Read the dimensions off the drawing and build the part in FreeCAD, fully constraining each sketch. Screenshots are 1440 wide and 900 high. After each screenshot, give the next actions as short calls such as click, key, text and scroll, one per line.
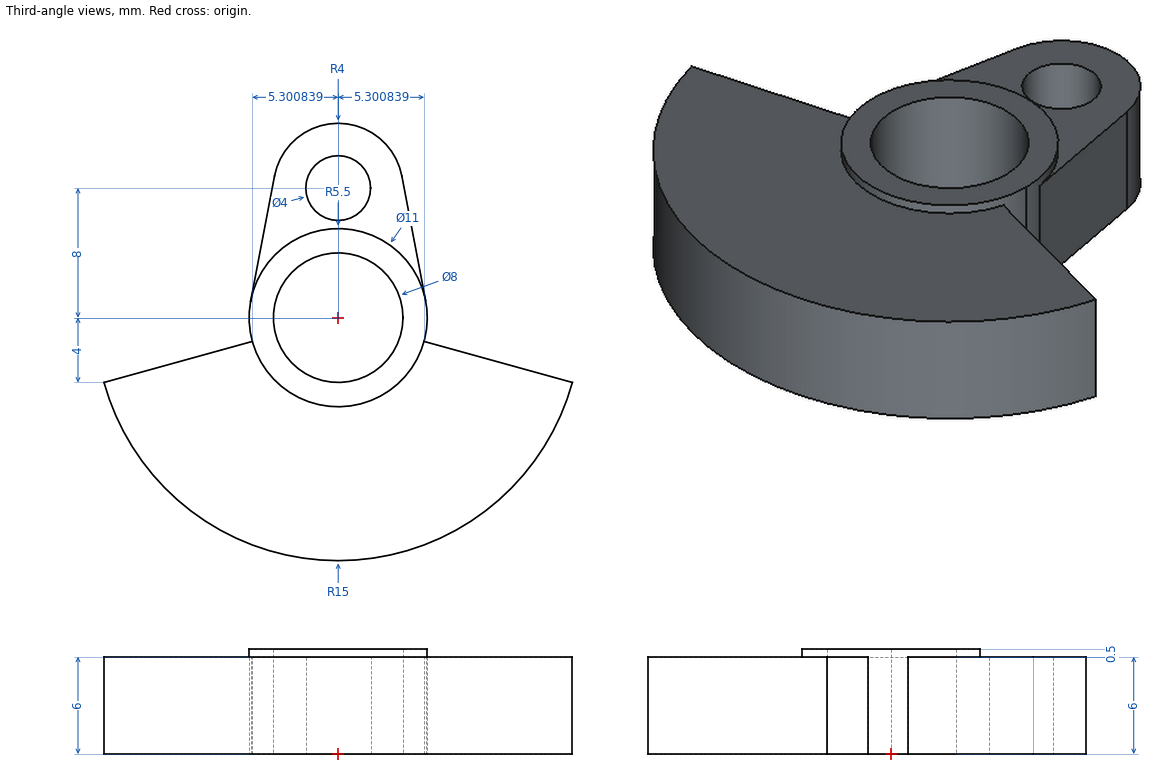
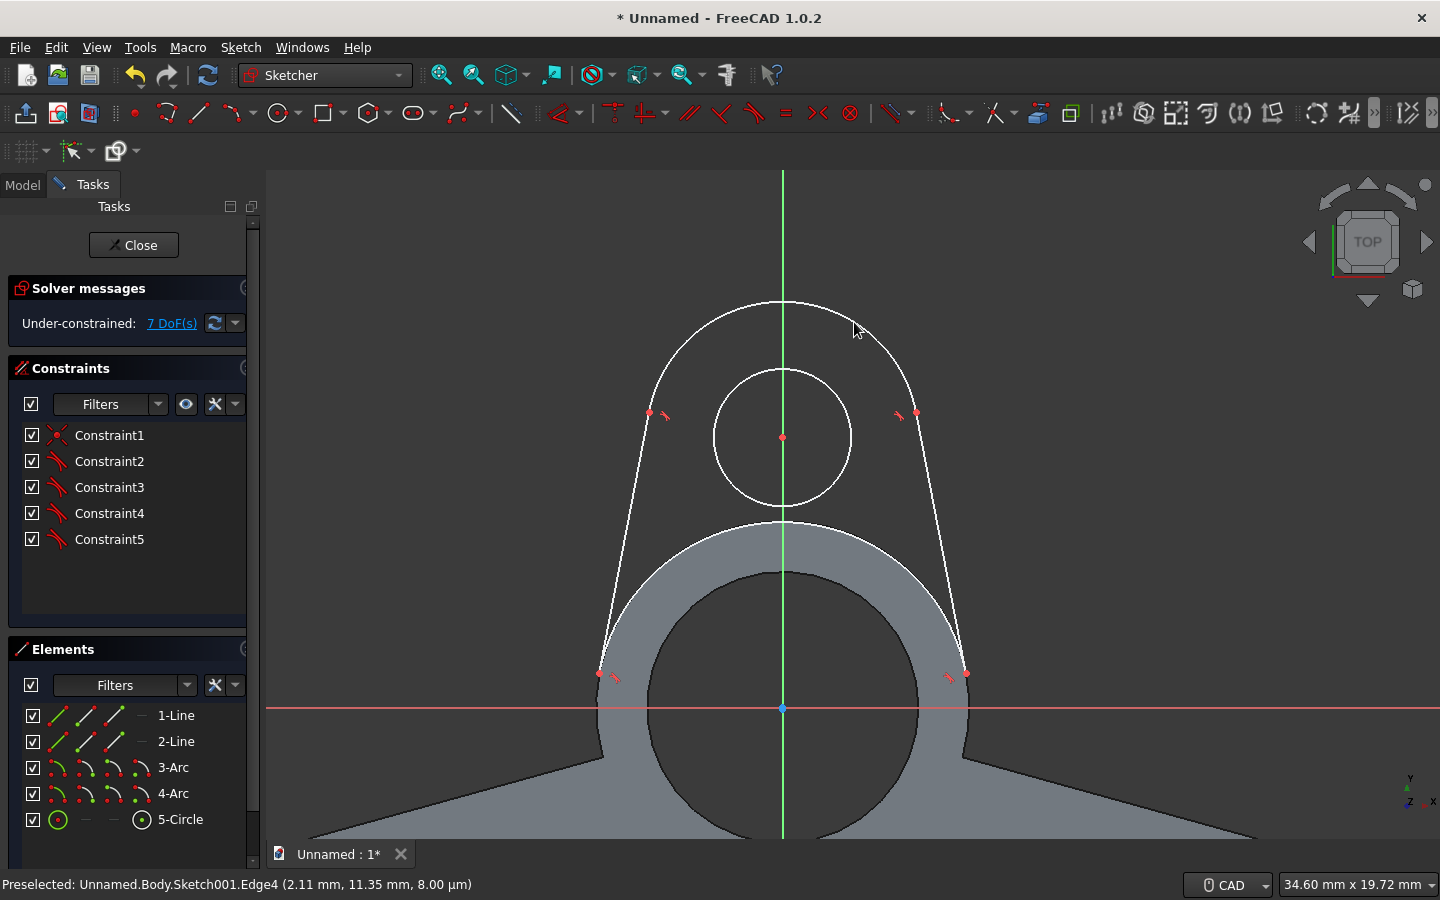
drag(772, 698, 793, 719)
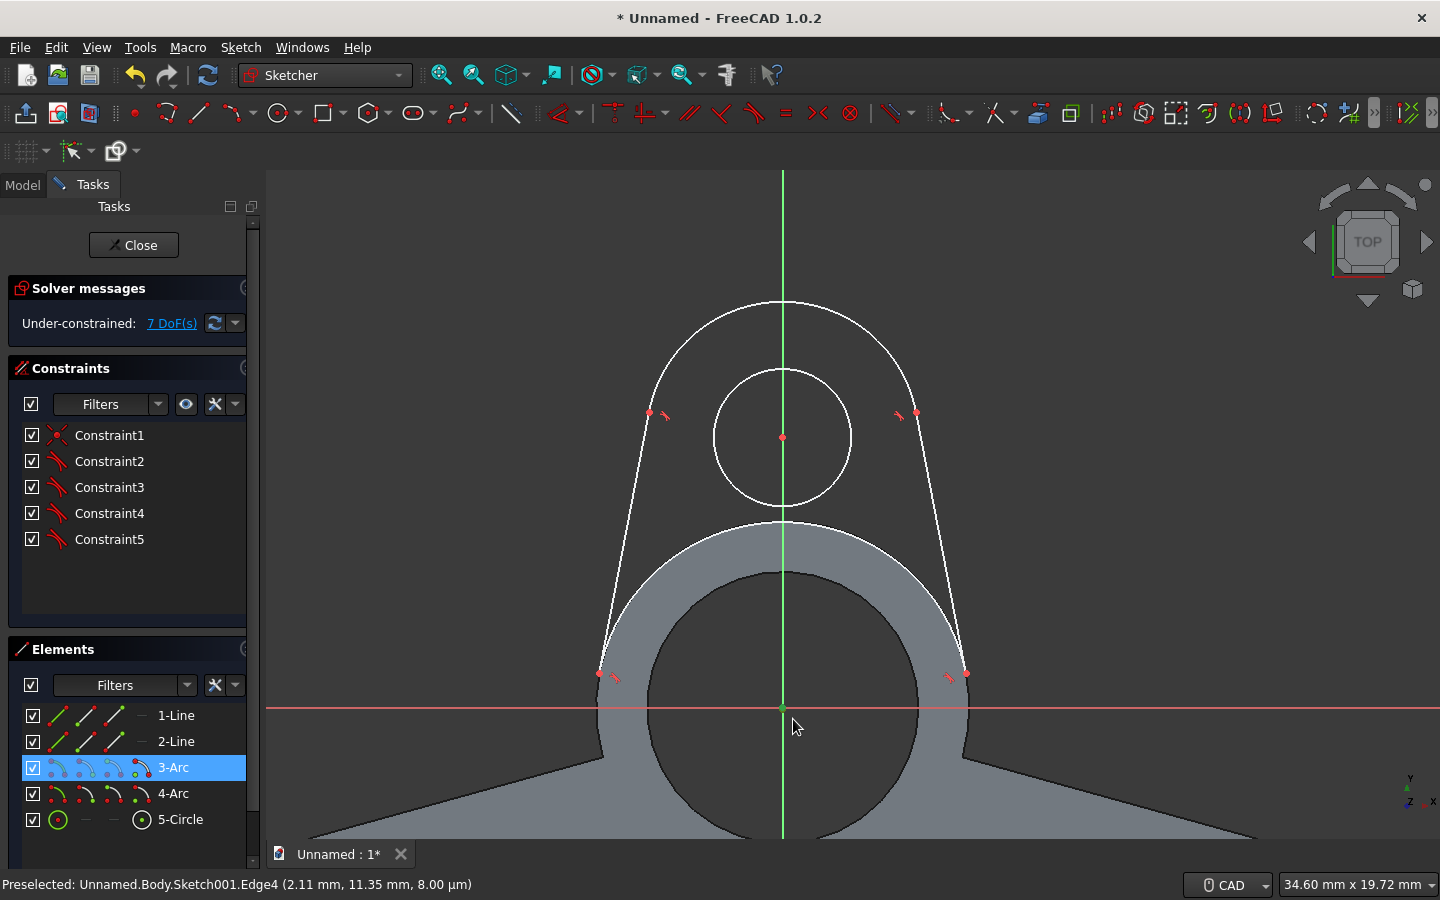
click(614, 114)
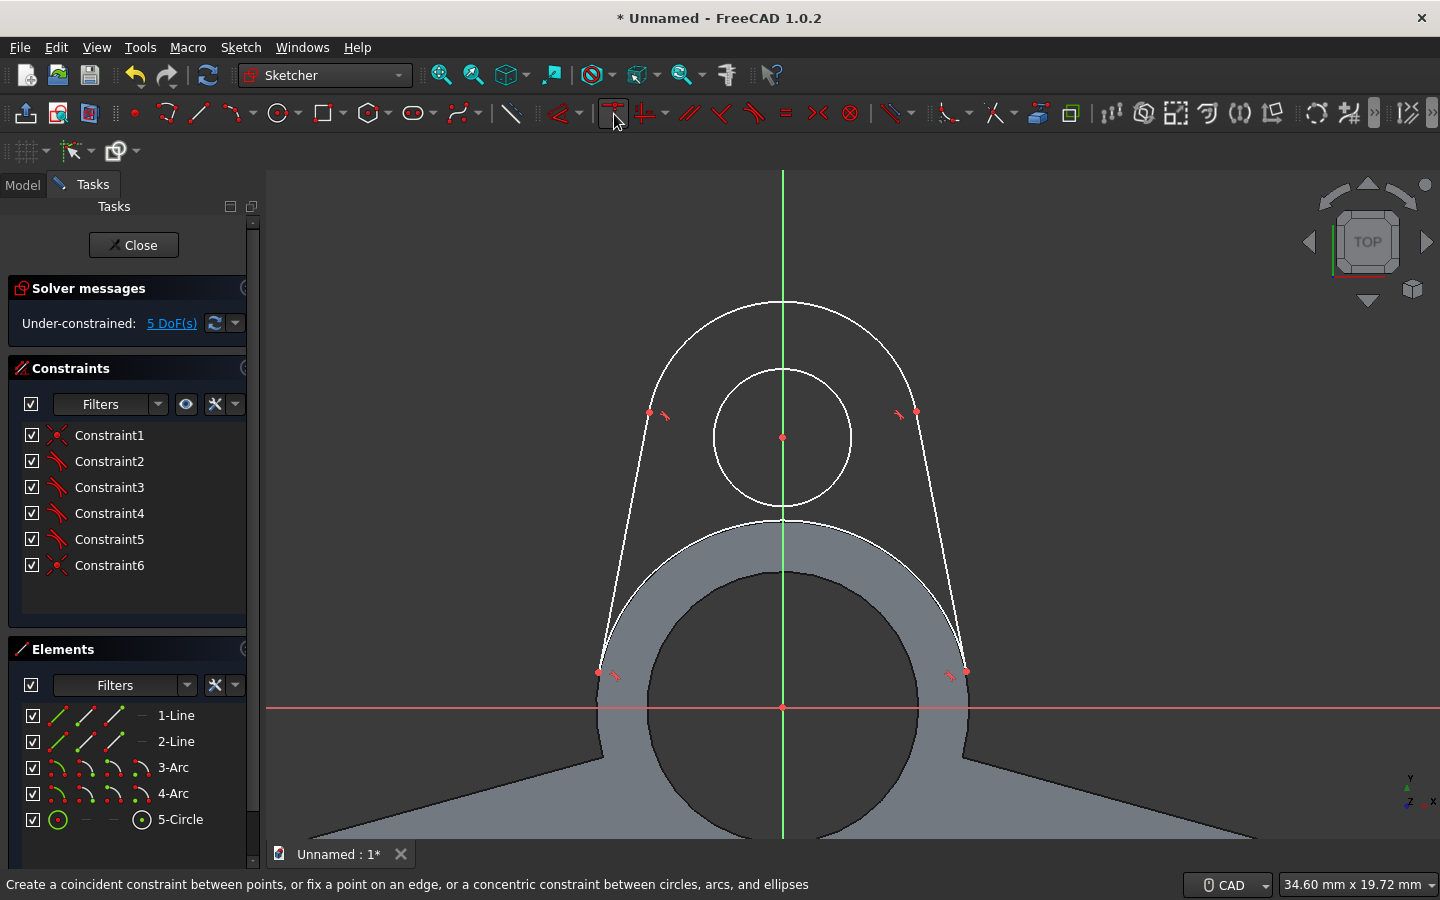
click(783, 438)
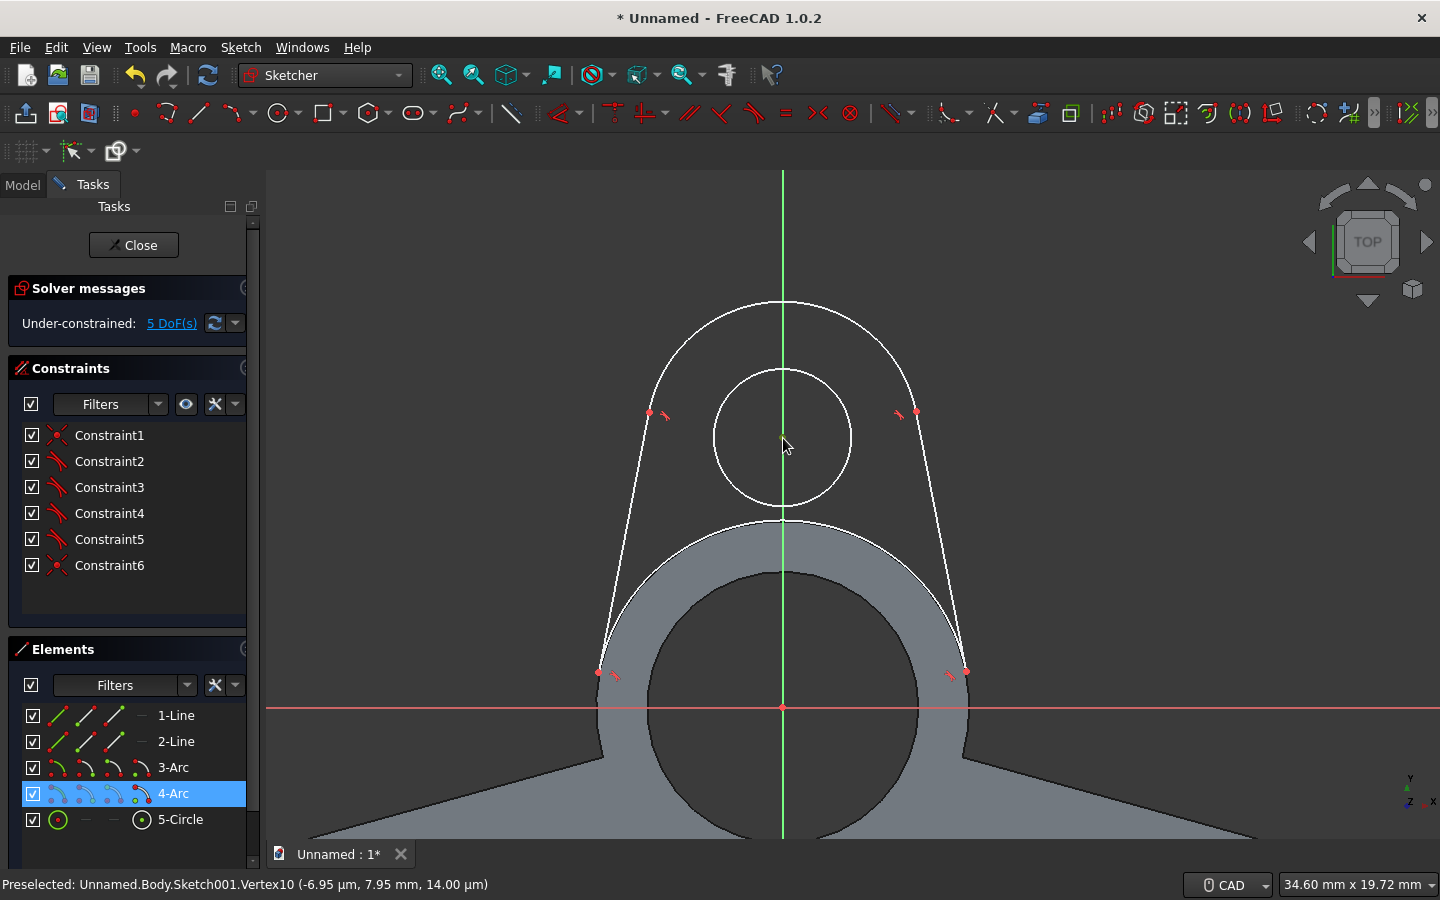
click(783, 767)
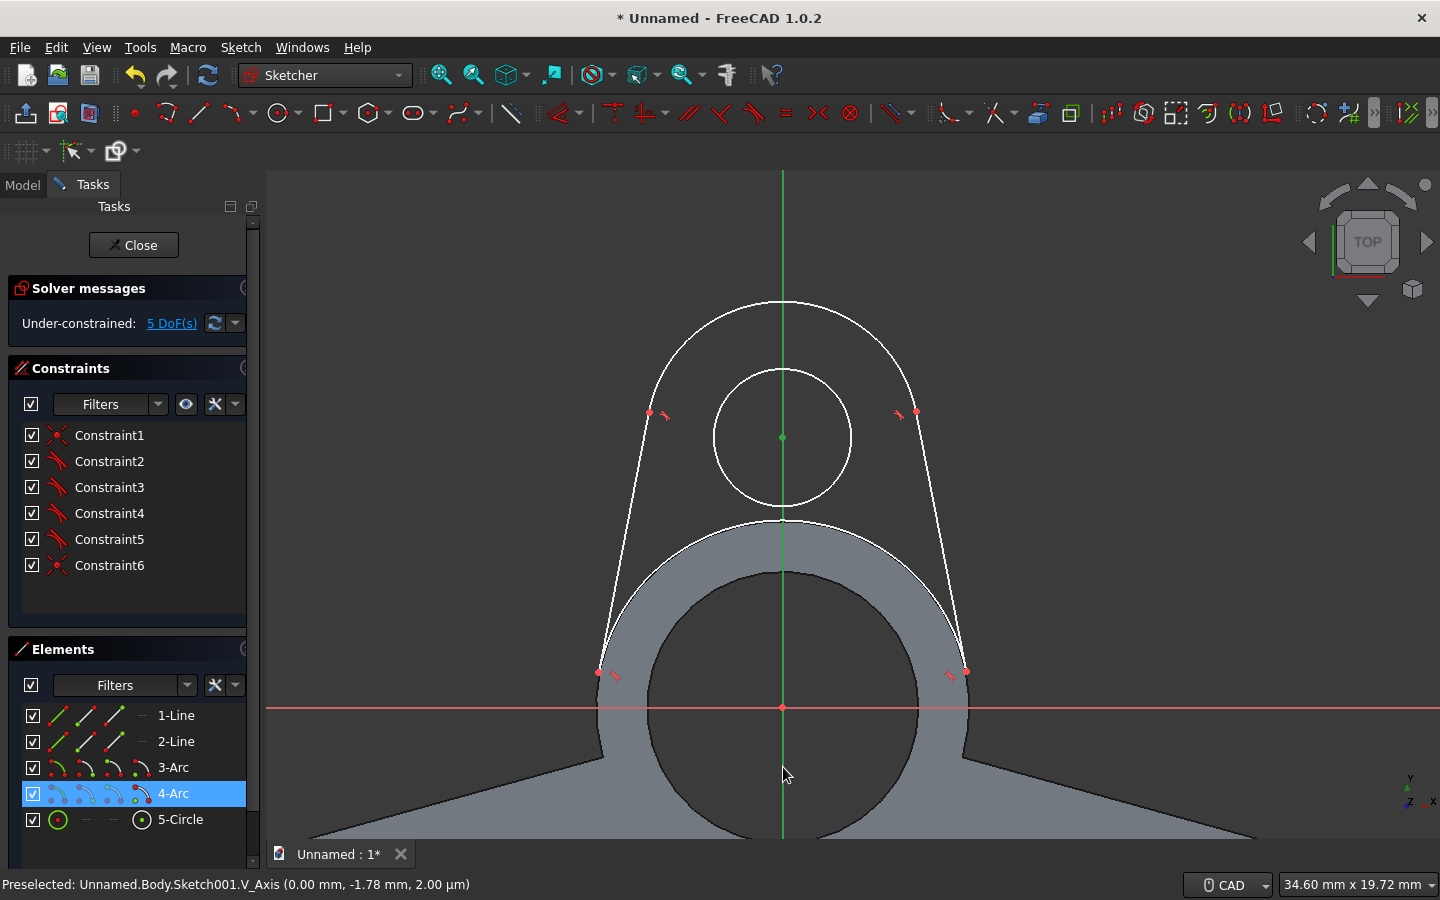
click(614, 114)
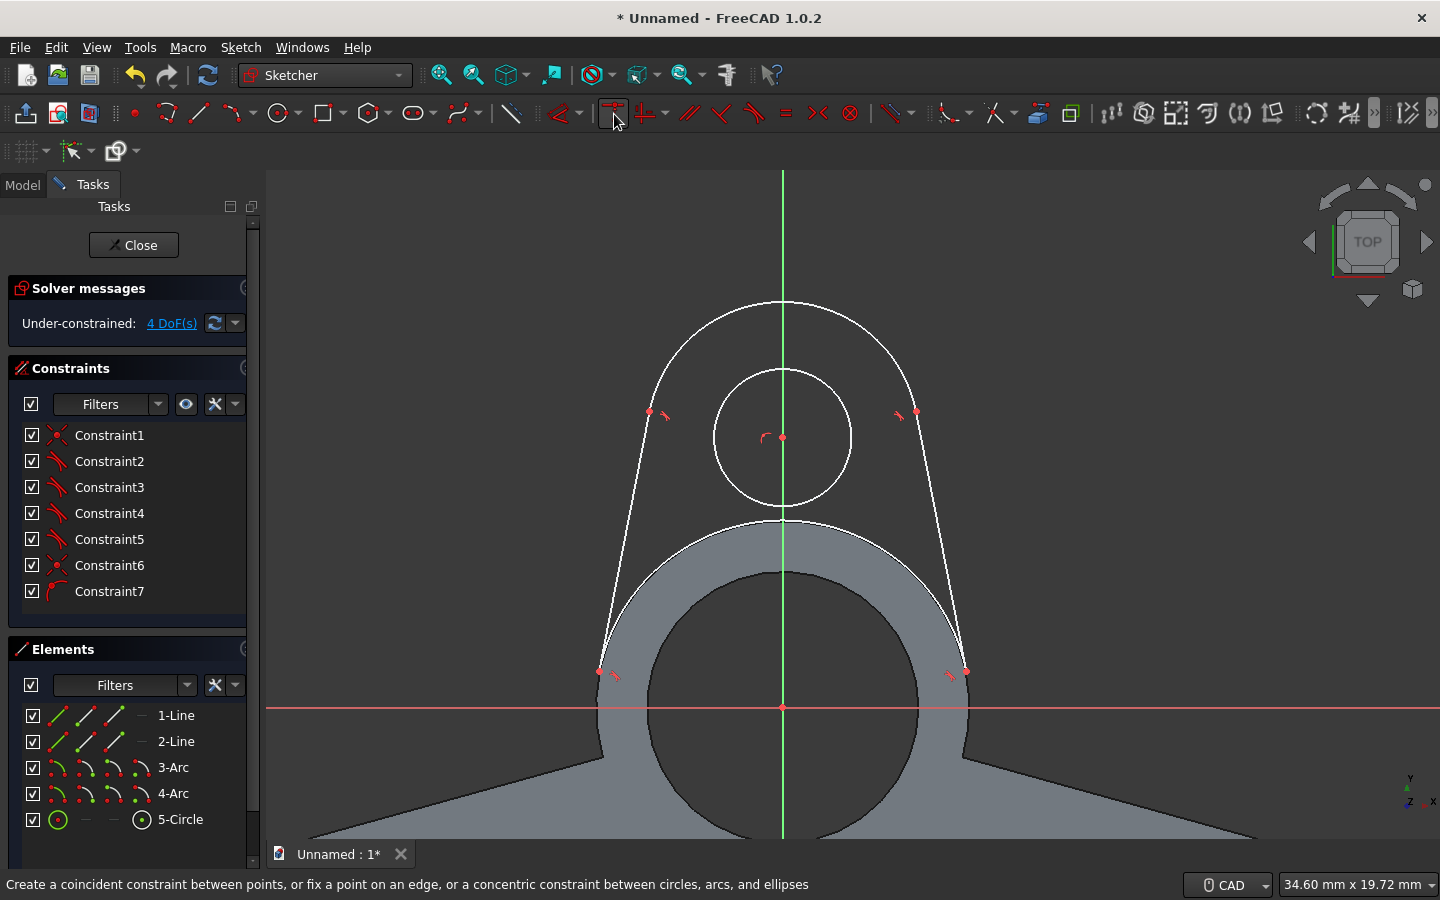
key(d)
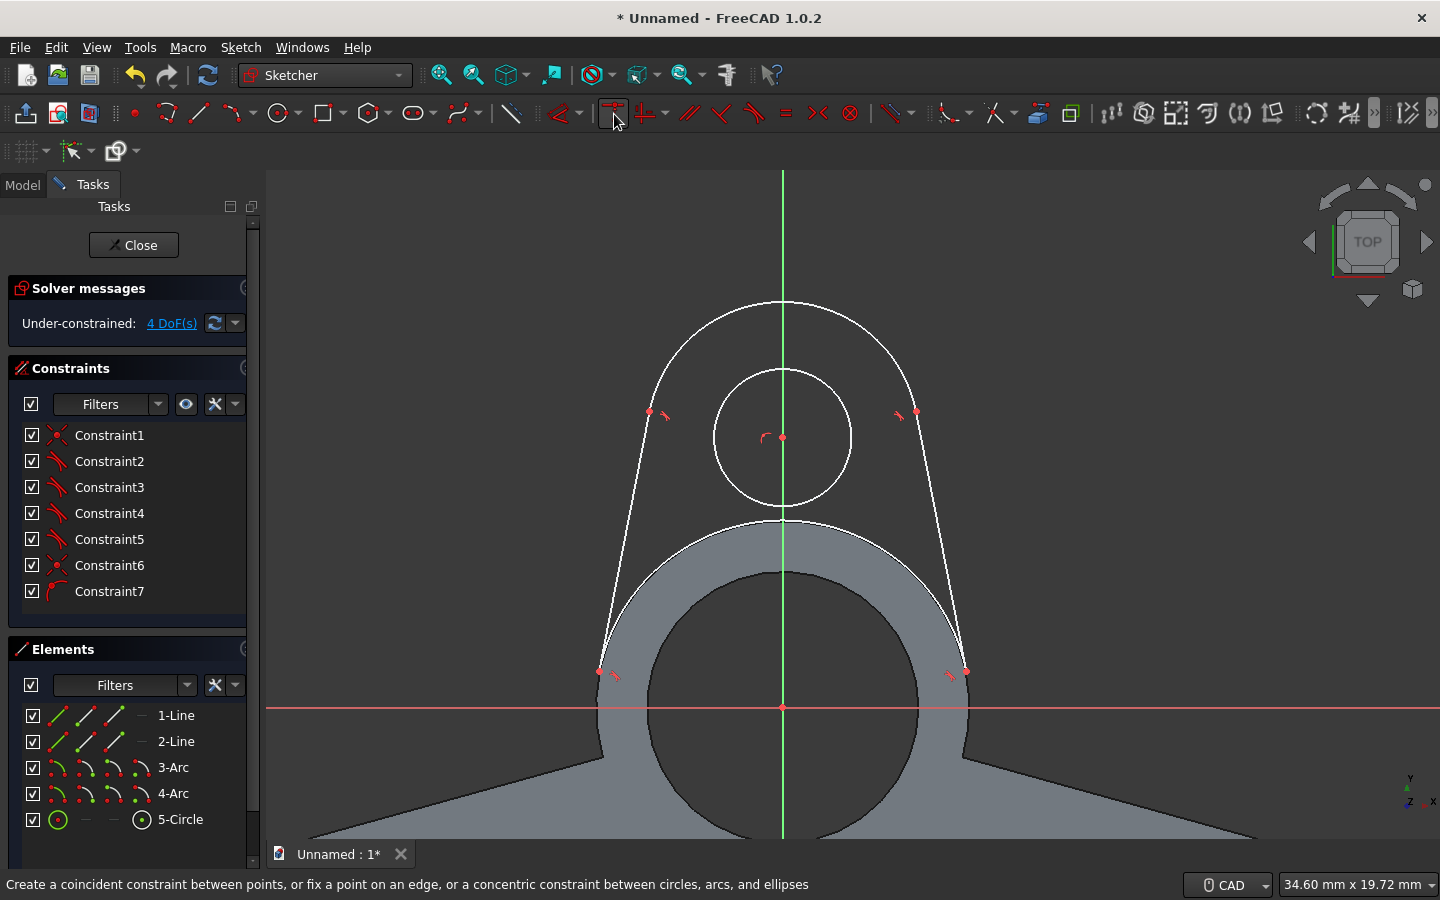
click(881, 548)
click(898, 521)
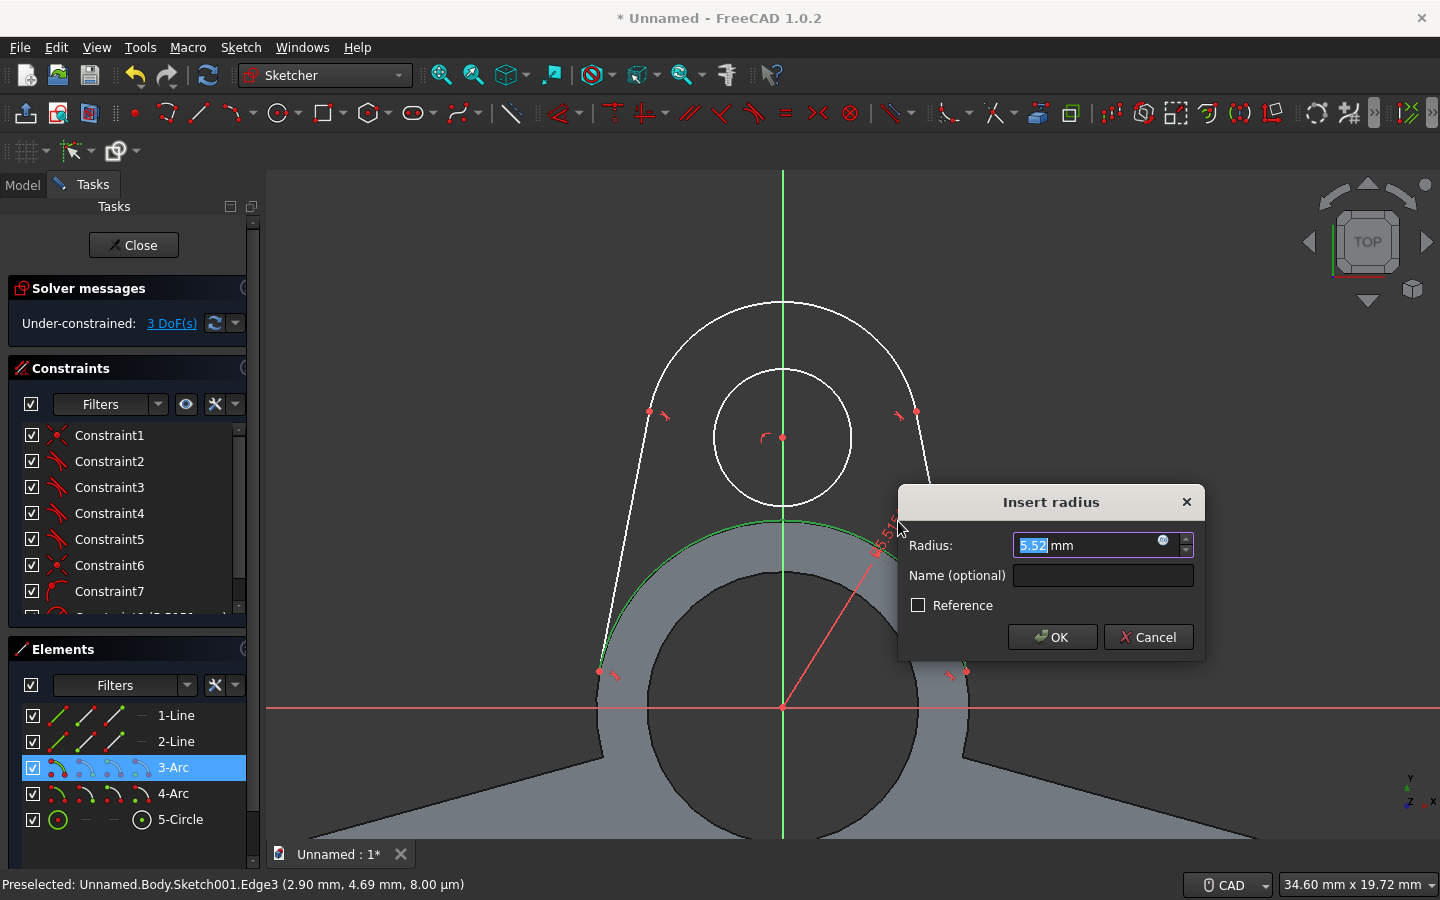
text(5.5)
key(Return)